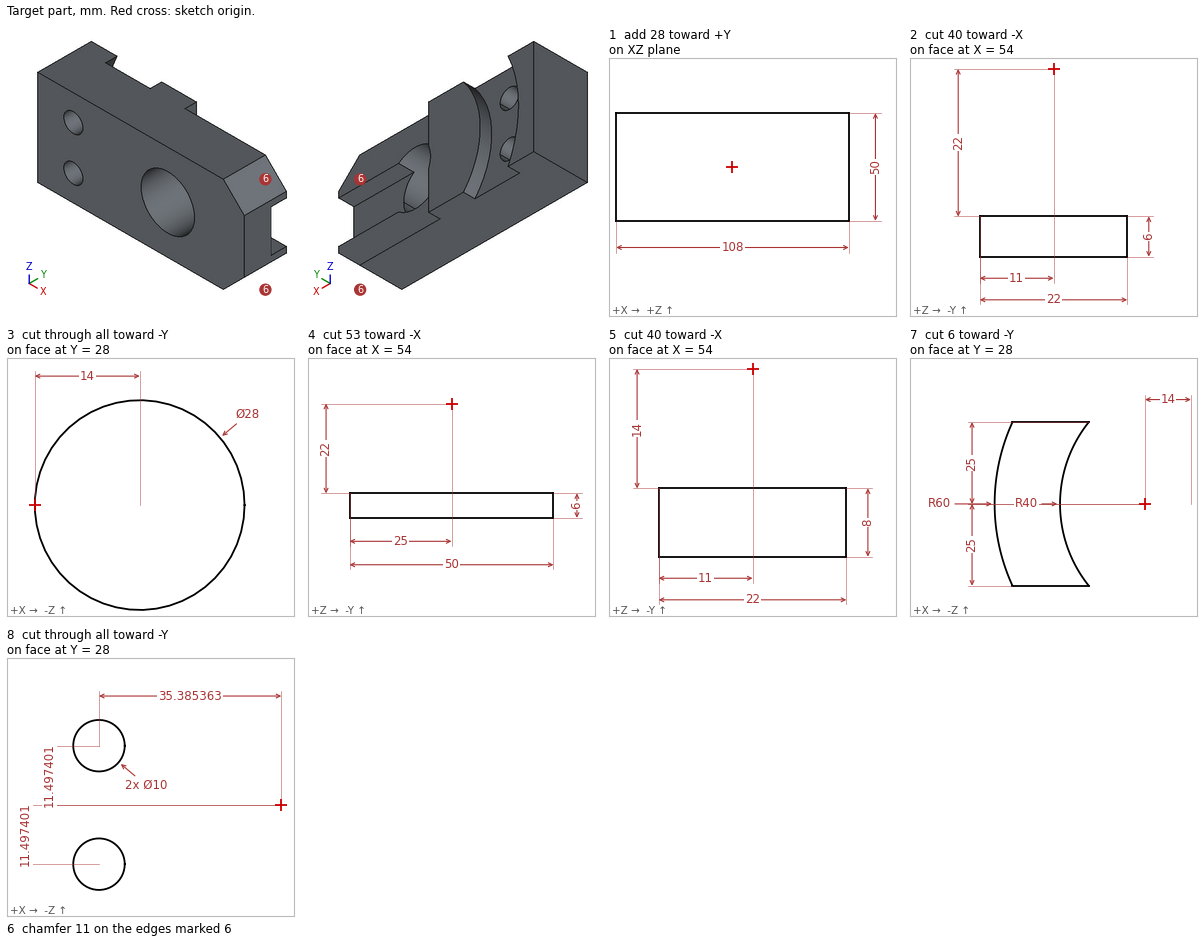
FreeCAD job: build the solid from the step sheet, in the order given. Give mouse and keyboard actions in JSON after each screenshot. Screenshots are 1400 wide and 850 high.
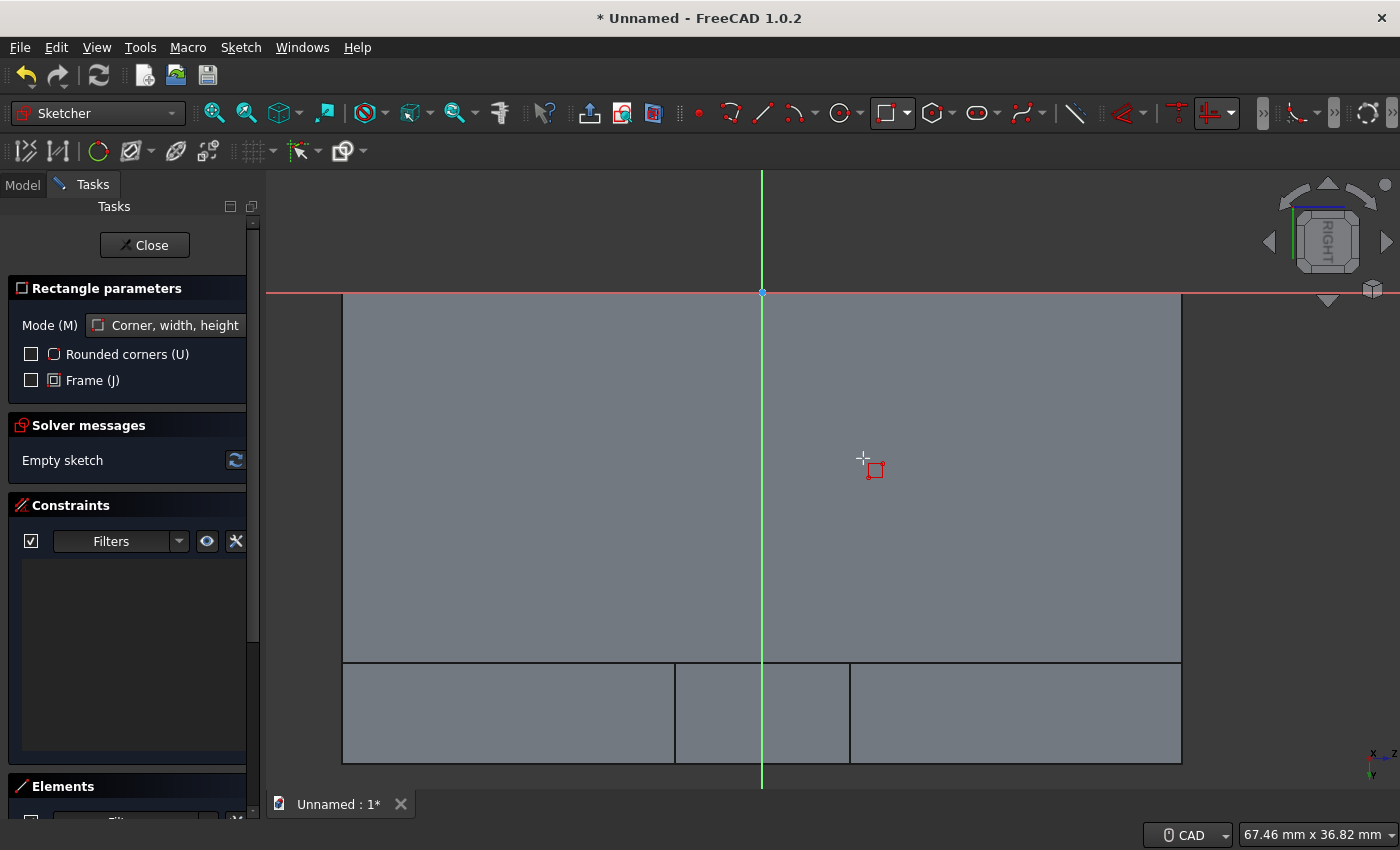
{"action": "left_click", "coordinate": [577, 528]}
{"action": "mouse_move", "coordinate": [947, 663]}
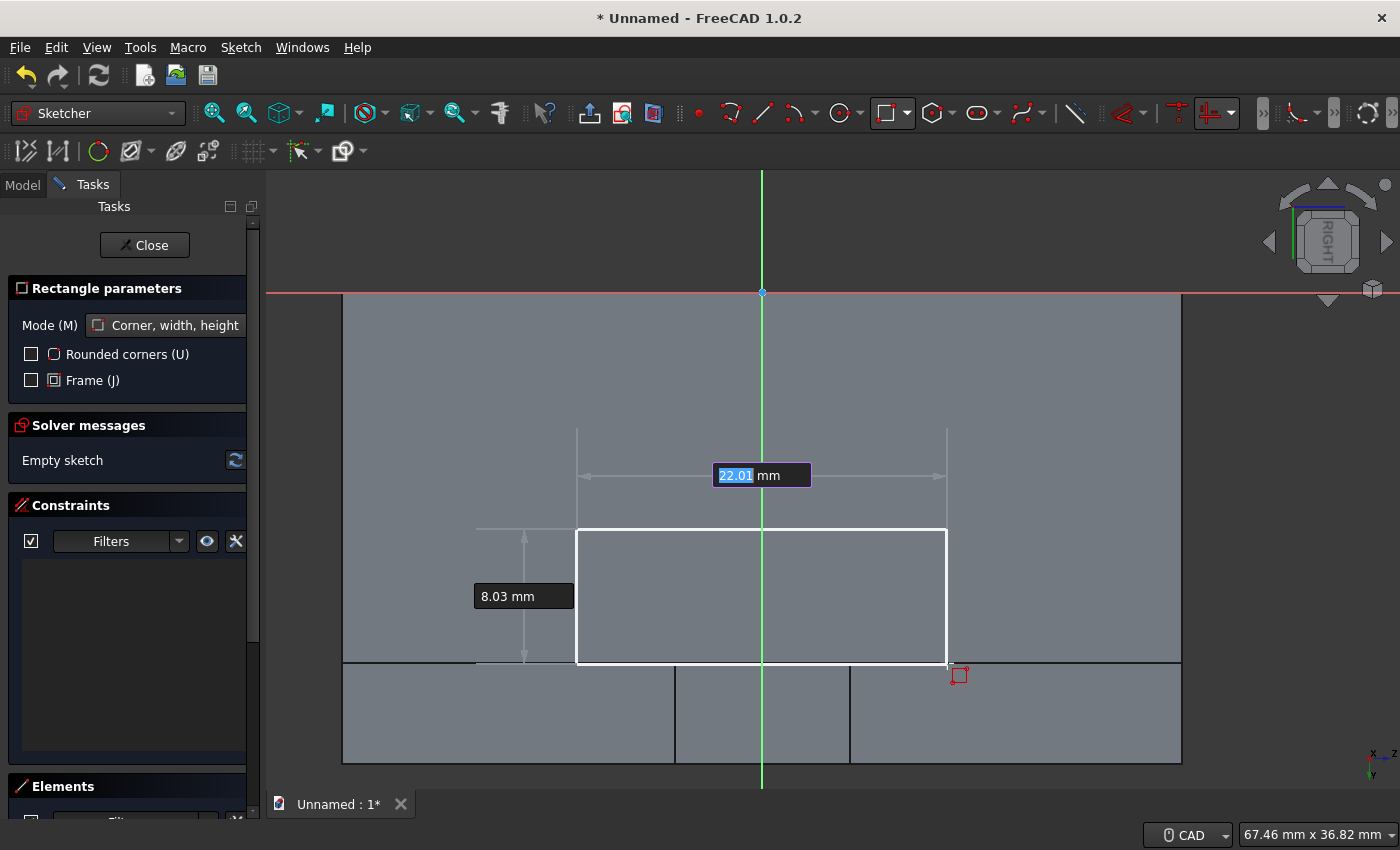
{"action": "type", "text": "22"}
{"action": "key", "text": "Tab"}
{"action": "type", "text": "8"}
{"action": "key", "text": "Return"}
{"action": "key", "text": "Escape"}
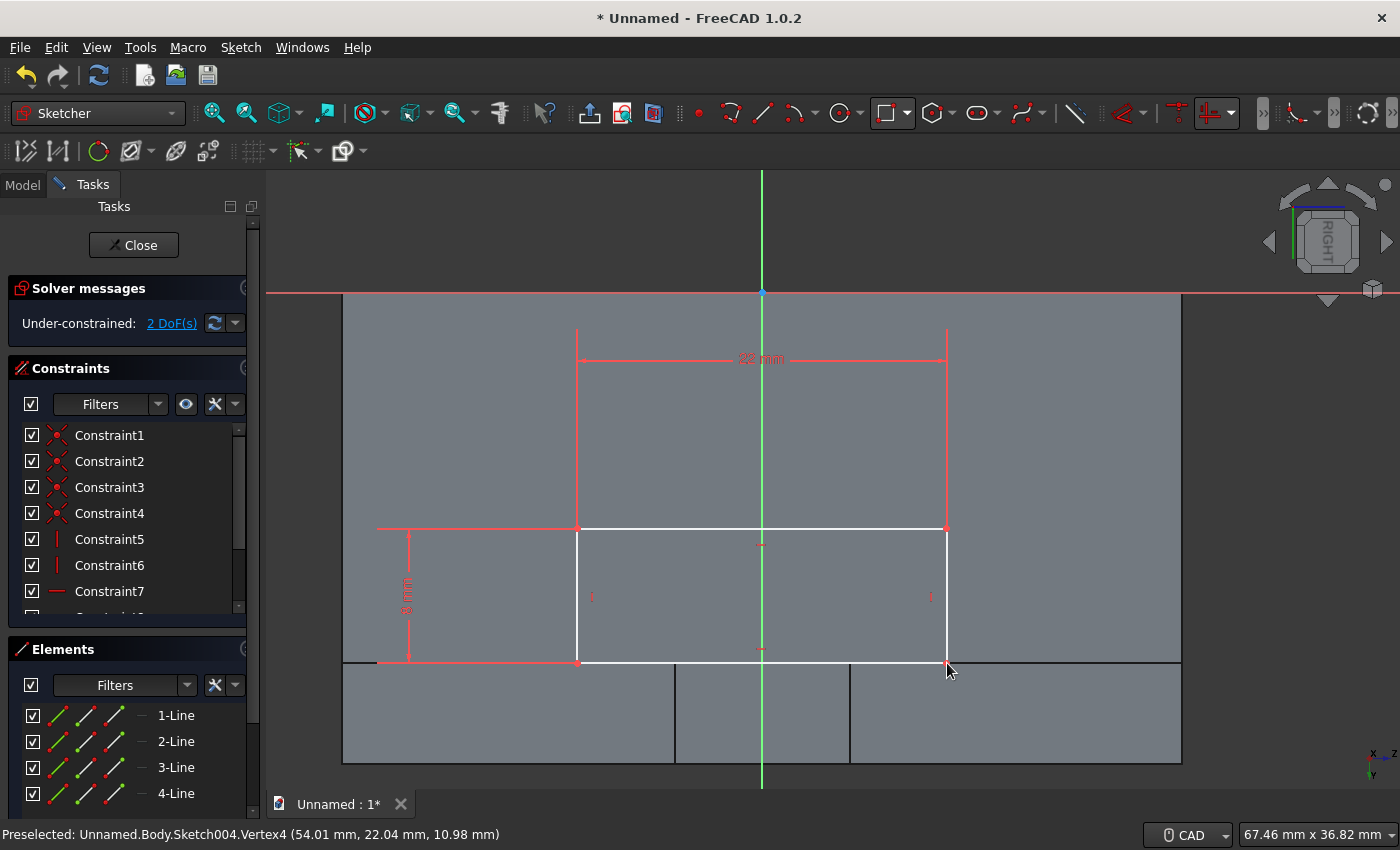
{"action": "key", "text": "d"}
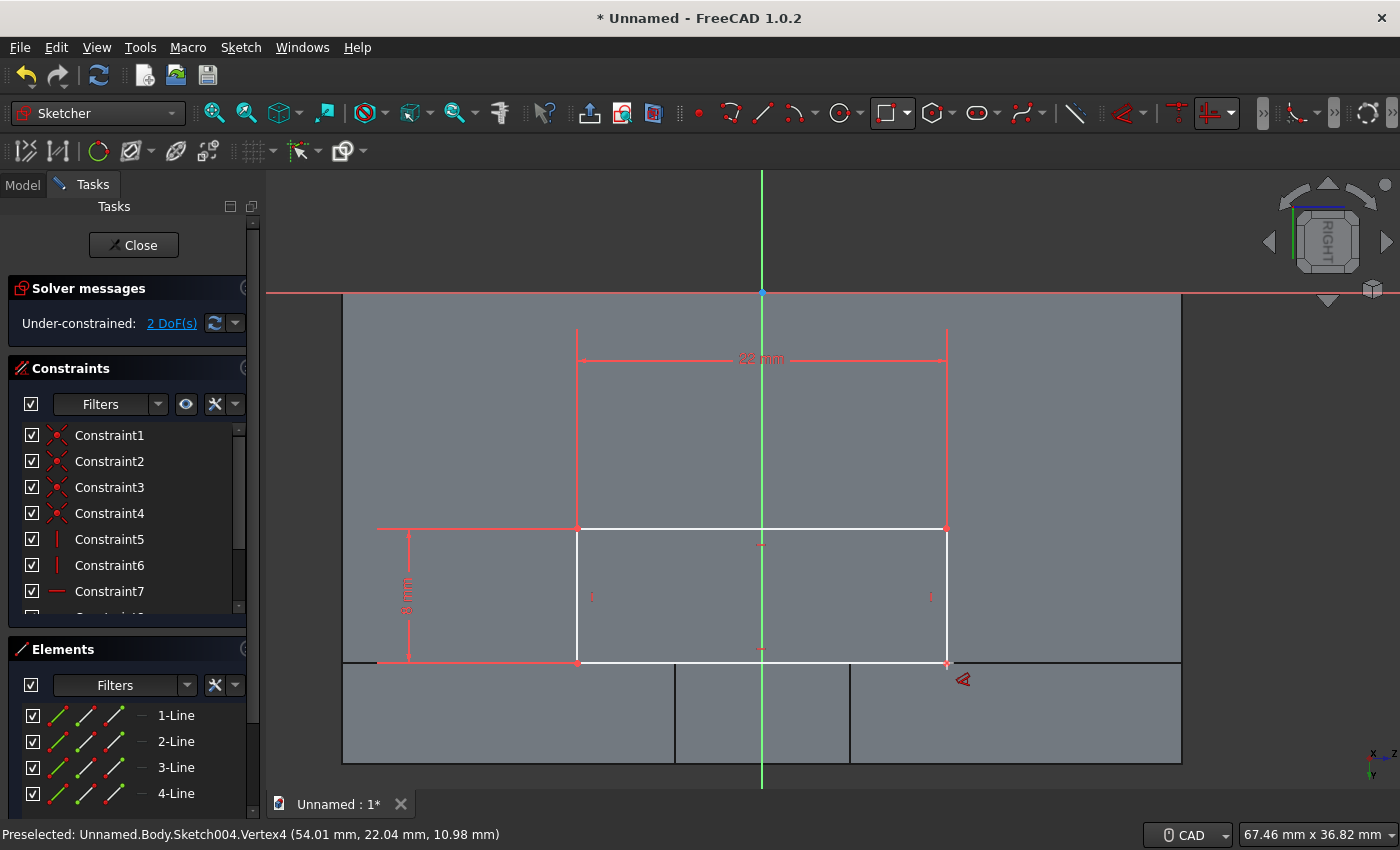
{"action": "left_click", "coordinate": [577, 529]}
{"action": "left_click", "coordinate": [670, 259]}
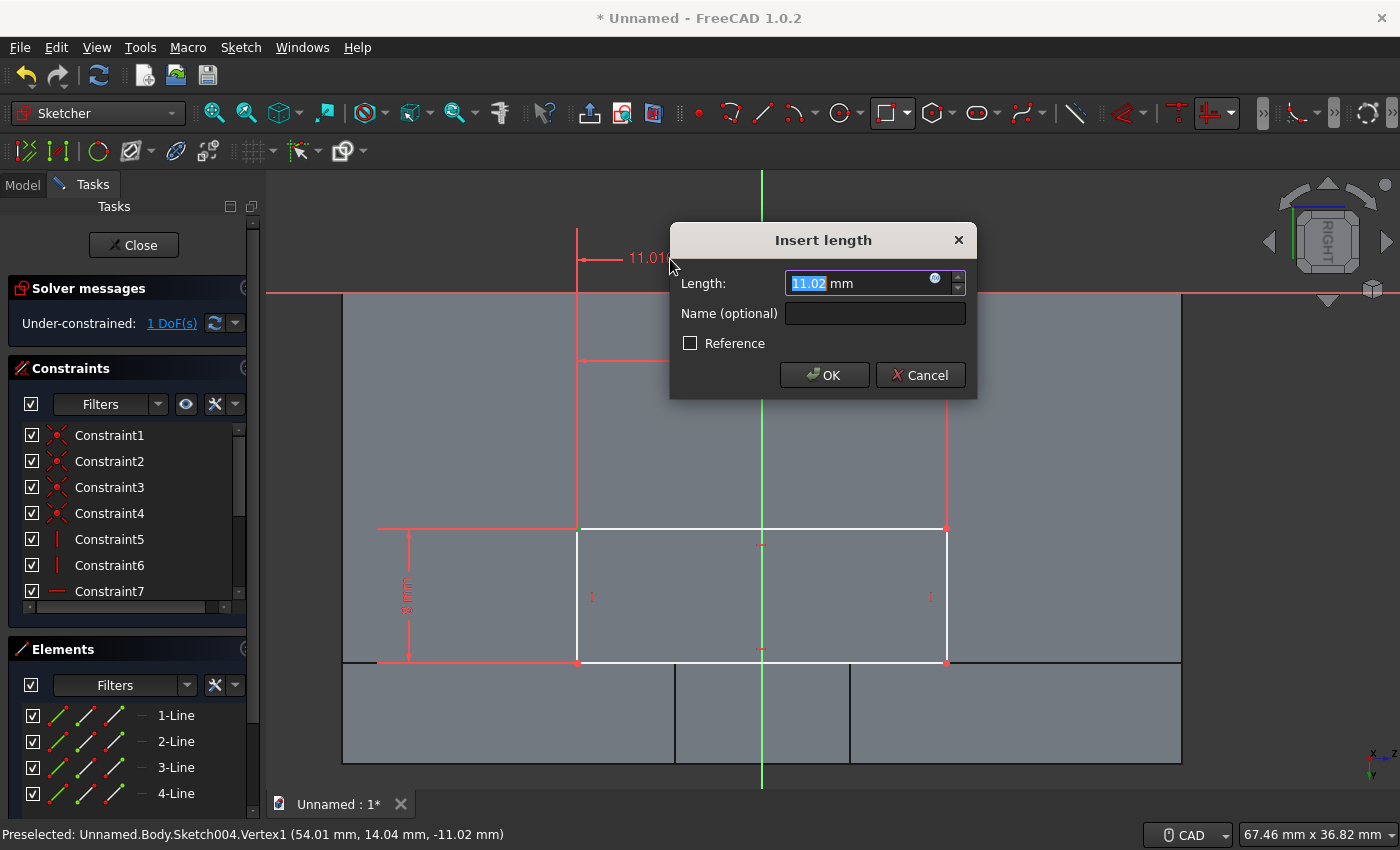
{"action": "type", "text": "11"}
{"action": "key", "text": "Return"}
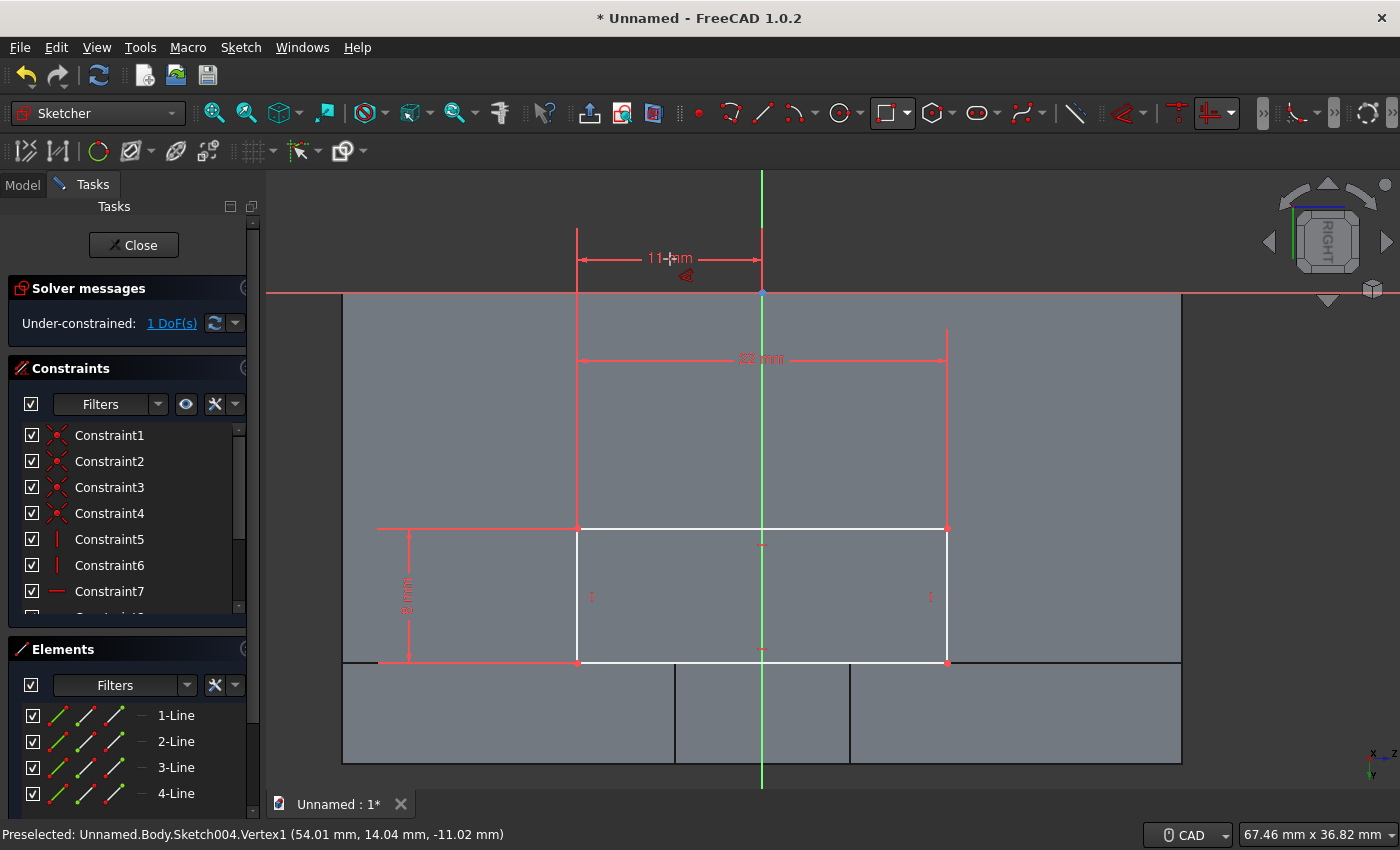
{"action": "left_click", "coordinate": [577, 529]}
{"action": "left_click", "coordinate": [543, 411]}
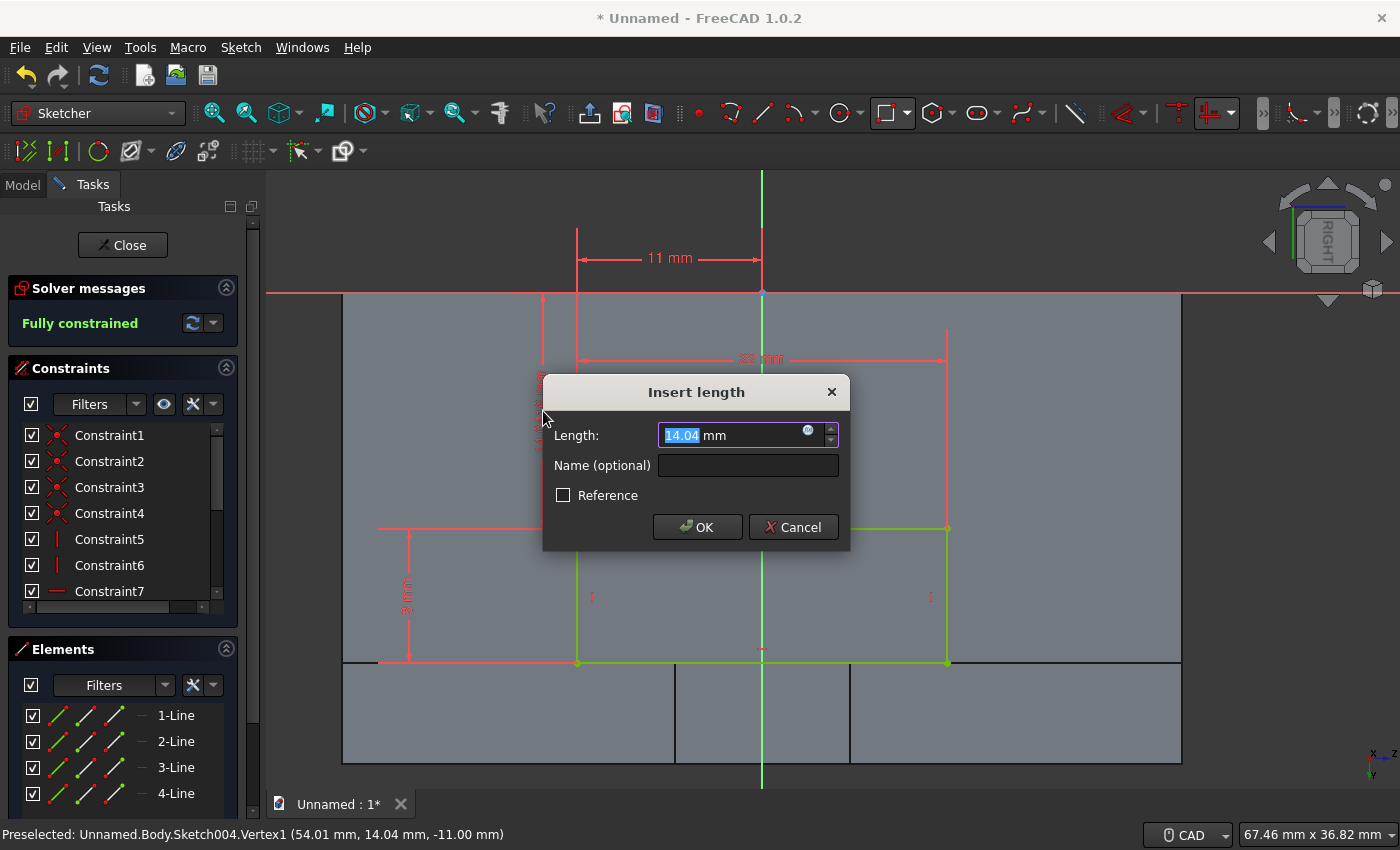
{"action": "type", "text": "14"}
{"action": "key", "text": "Return"}
{"action": "key", "text": "Escape"}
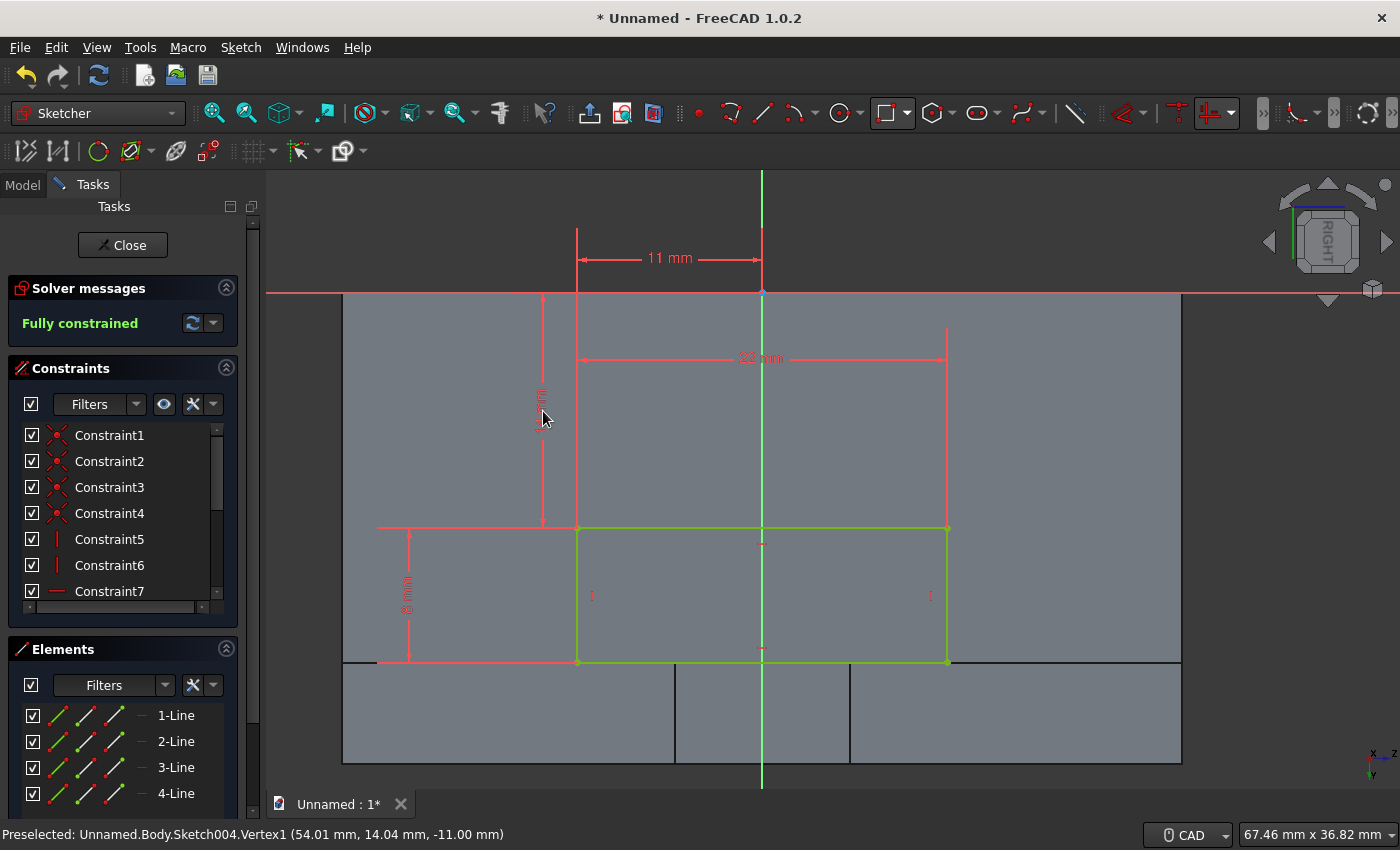
{"action": "left_click", "coordinate": [123, 245]}